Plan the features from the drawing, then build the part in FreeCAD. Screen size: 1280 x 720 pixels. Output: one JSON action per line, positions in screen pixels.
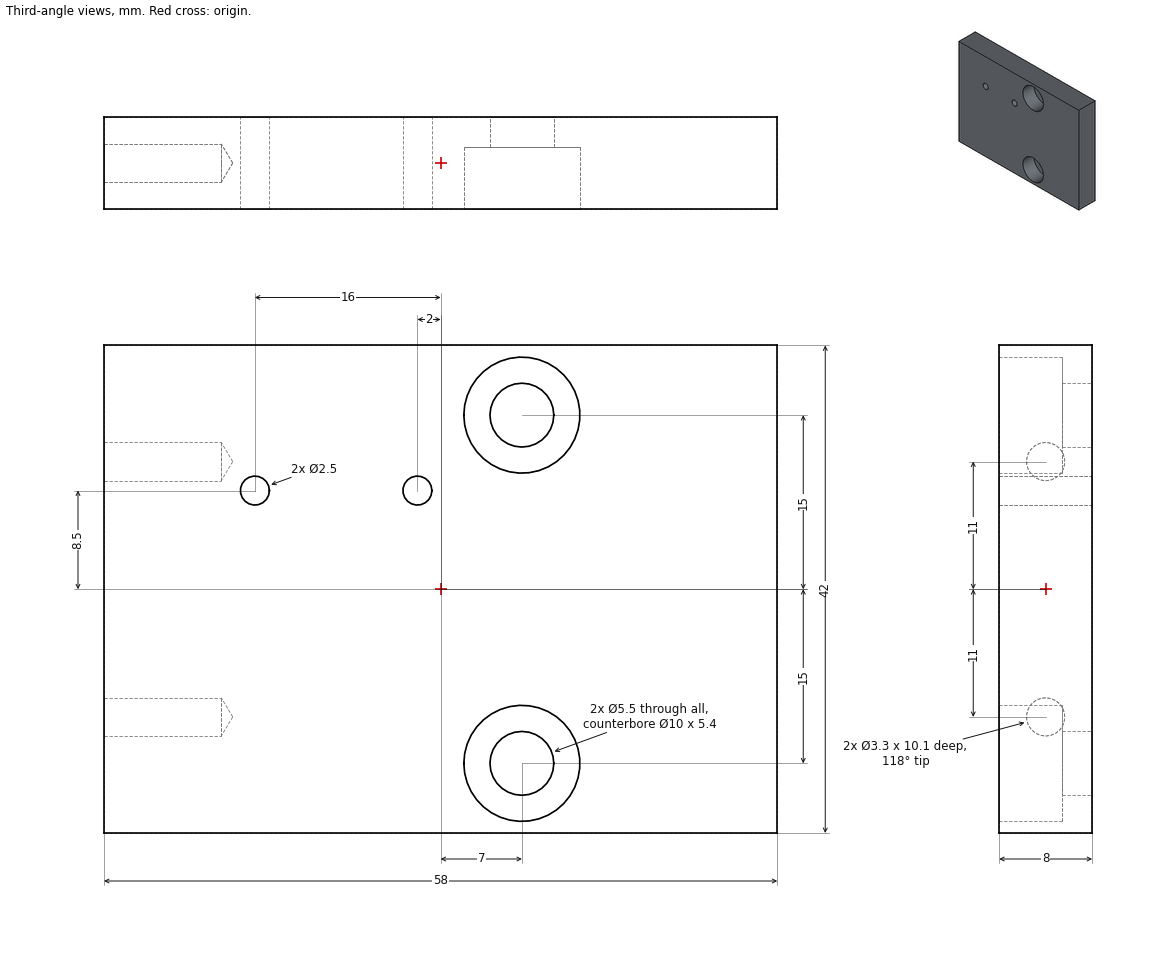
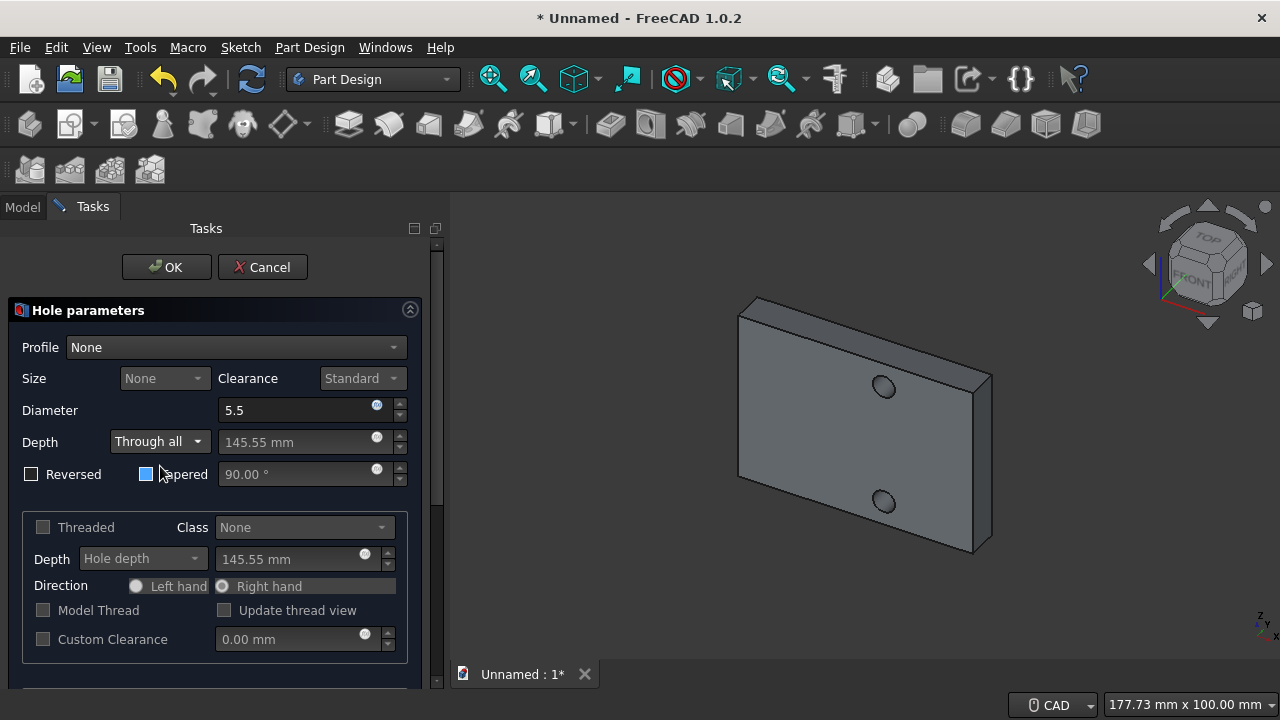
{"action": "scroll", "coordinate": [437, 463], "scroll_direction": "down", "scroll_amount": 2}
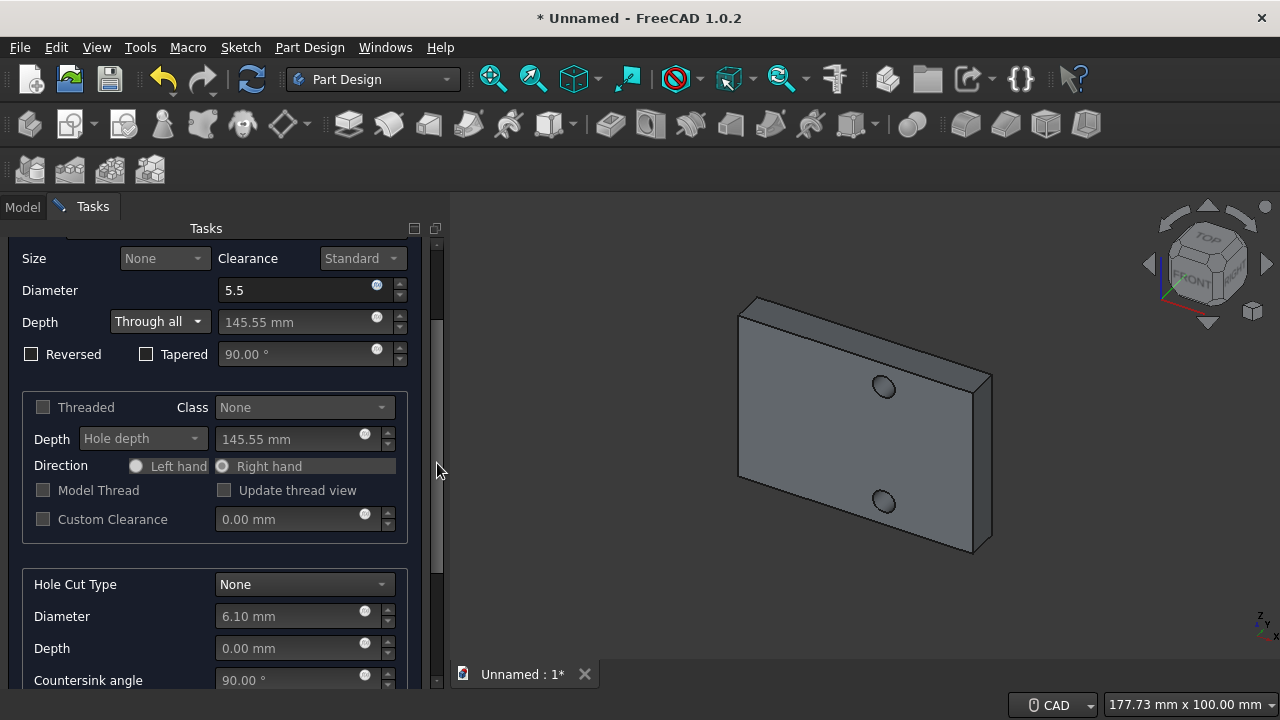
{"action": "left_click", "coordinate": [306, 584]}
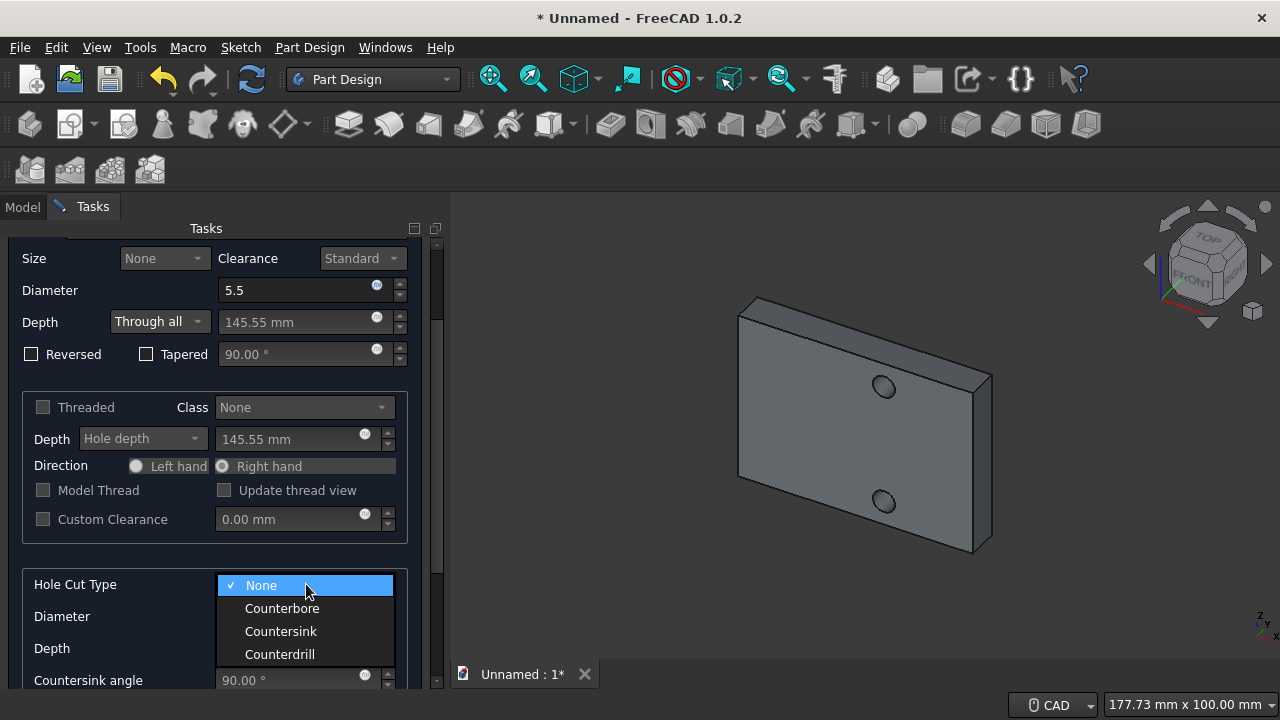
{"action": "left_click", "coordinate": [304, 608]}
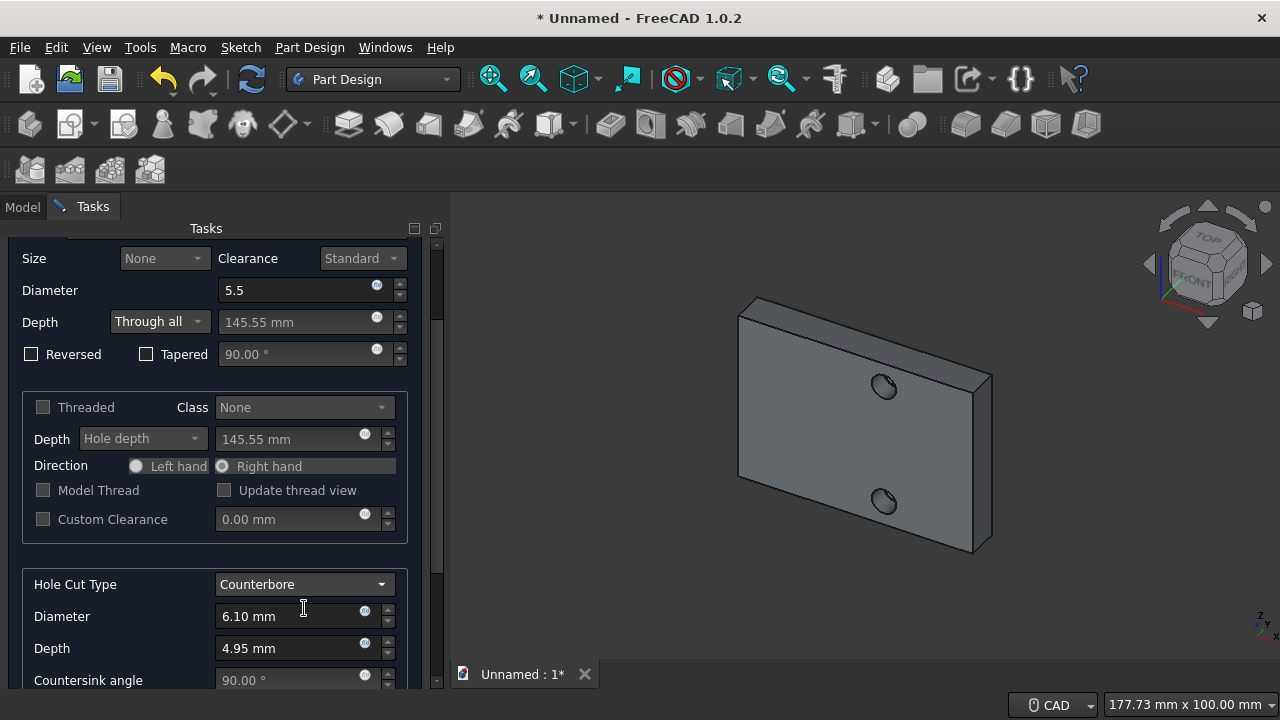
{"action": "triple_click", "coordinate": [298, 616]}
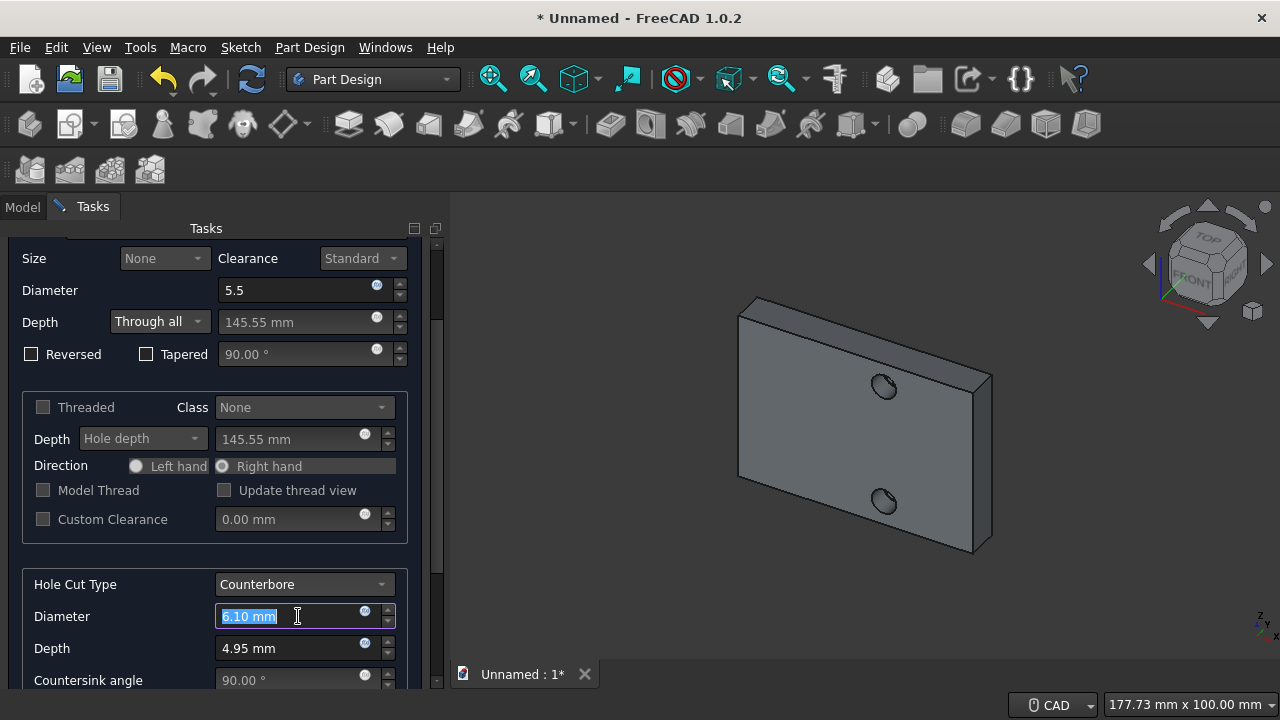
{"action": "type", "text": "10"}
{"action": "key", "text": "Tab"}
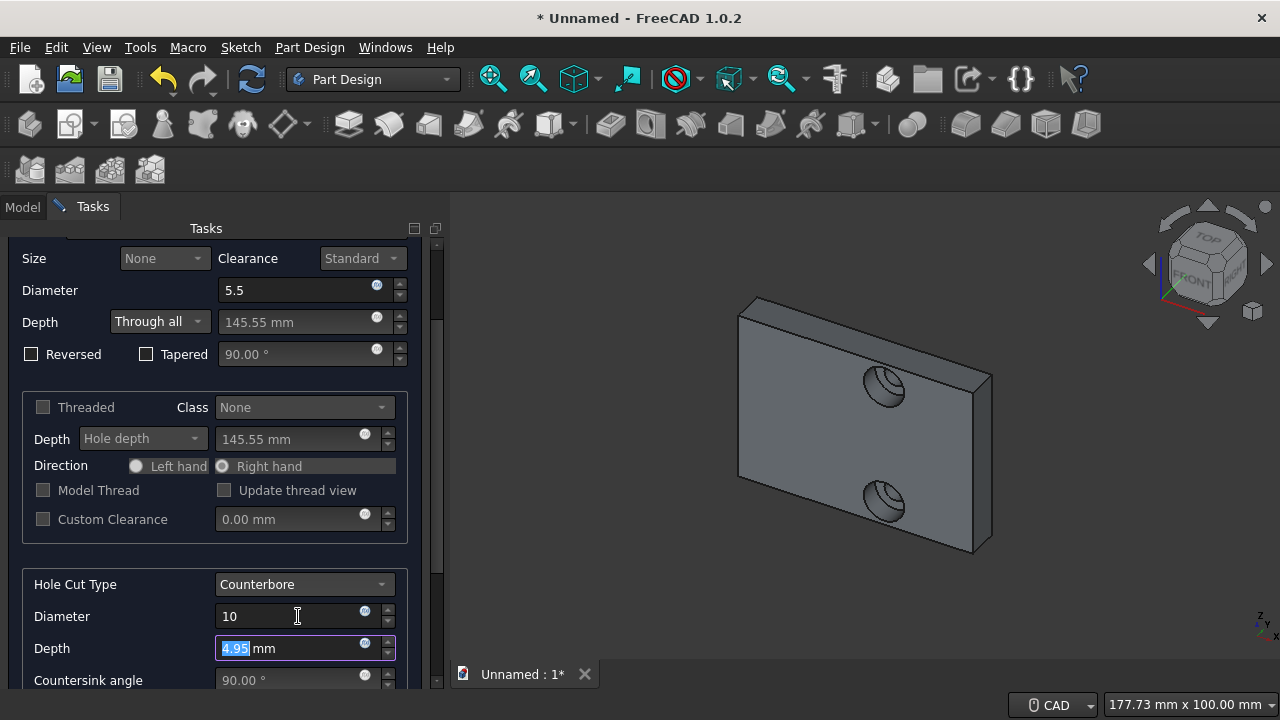
{"action": "type", "text": "5.4"}
{"action": "key", "text": "Tab"}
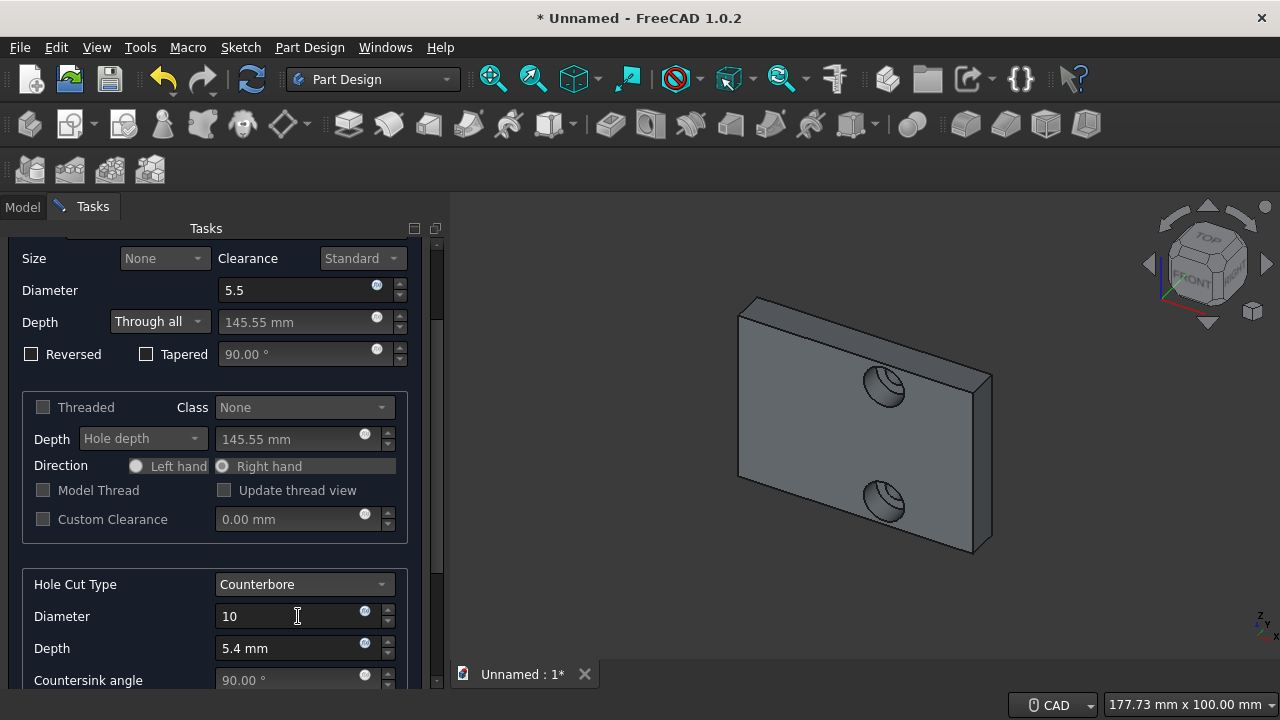
{"action": "scroll", "coordinate": [437, 463], "scroll_direction": "up", "scroll_amount": 3}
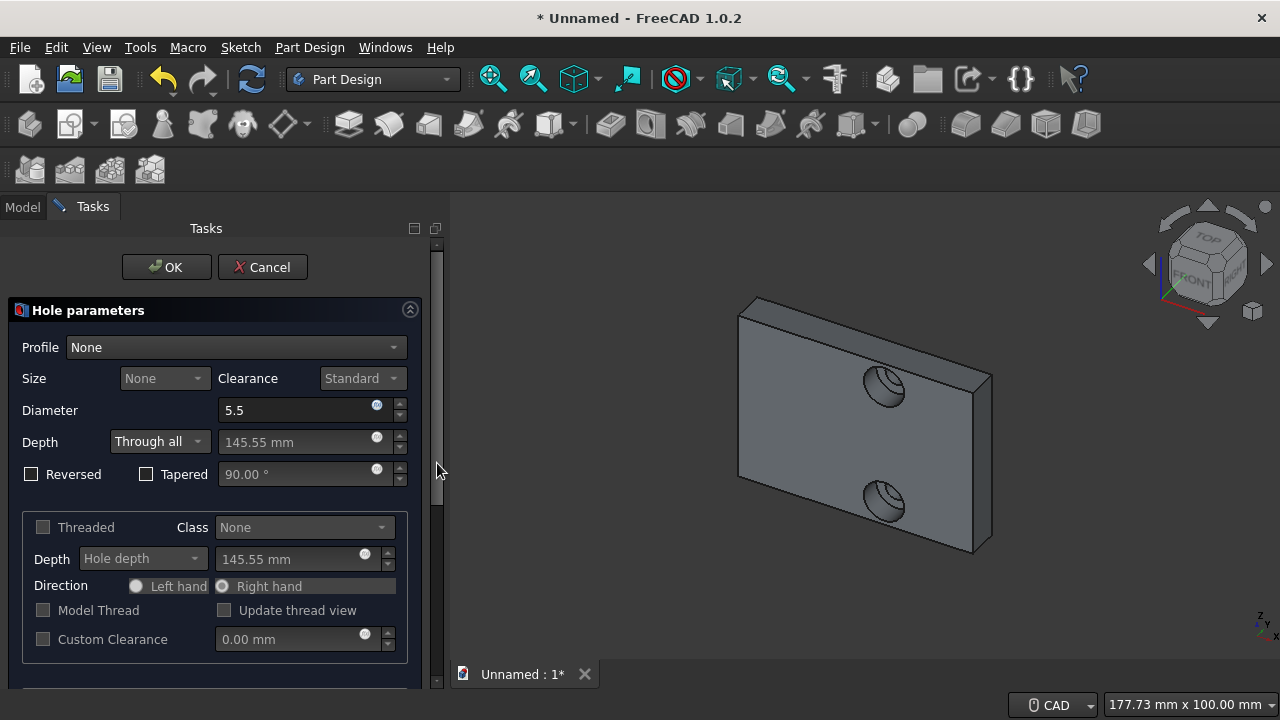
{"action": "left_click", "coordinate": [167, 267]}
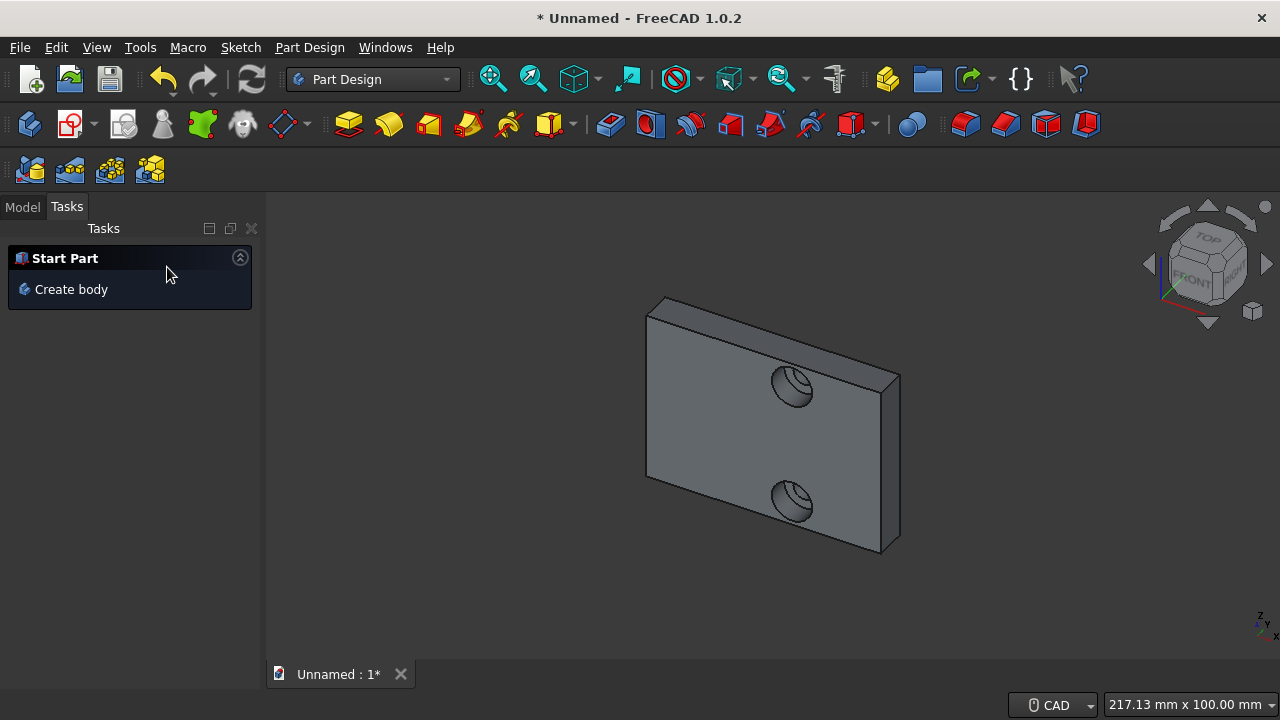
{"action": "key", "text": "6"}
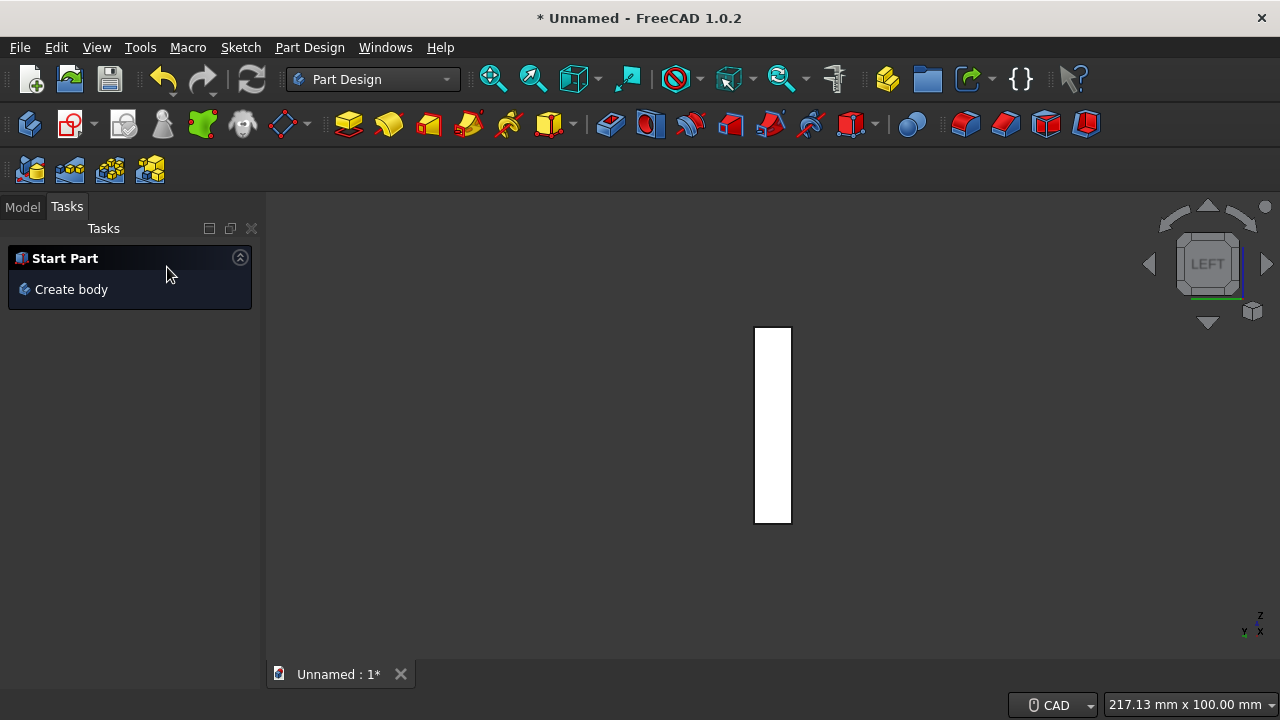
{"action": "key", "text": "v f"}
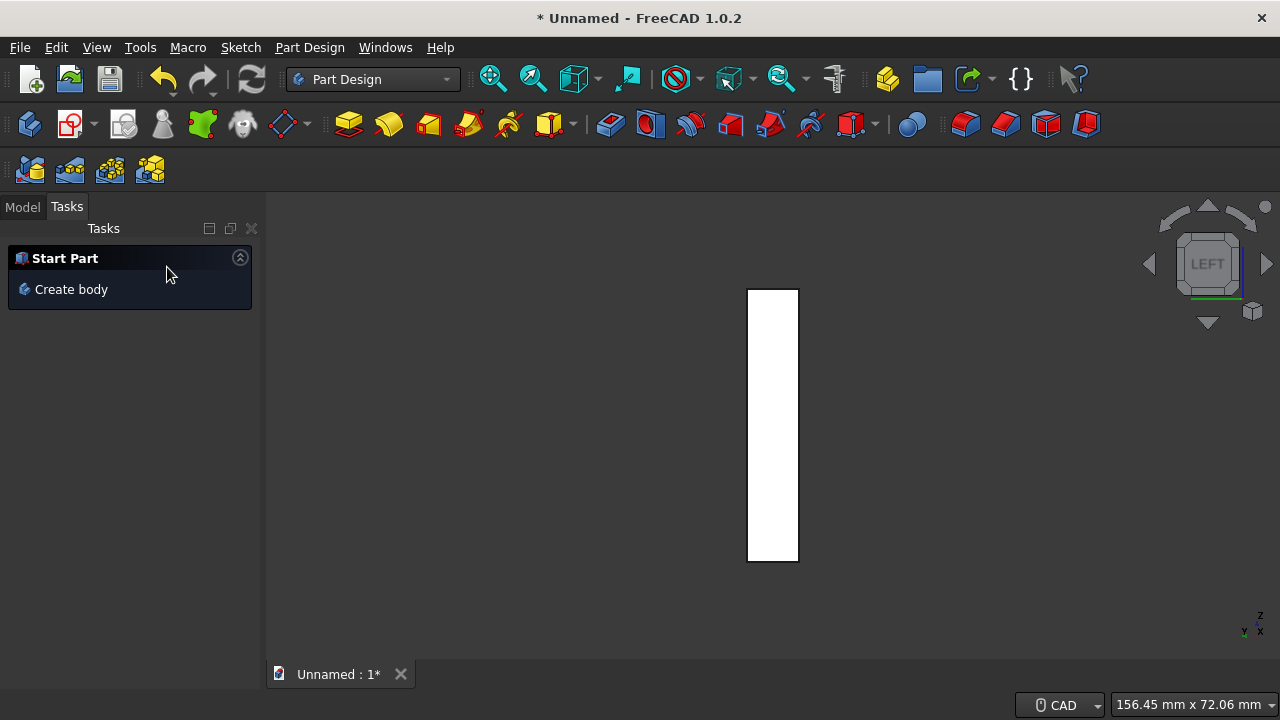
{"action": "left_click", "coordinate": [773, 347]}